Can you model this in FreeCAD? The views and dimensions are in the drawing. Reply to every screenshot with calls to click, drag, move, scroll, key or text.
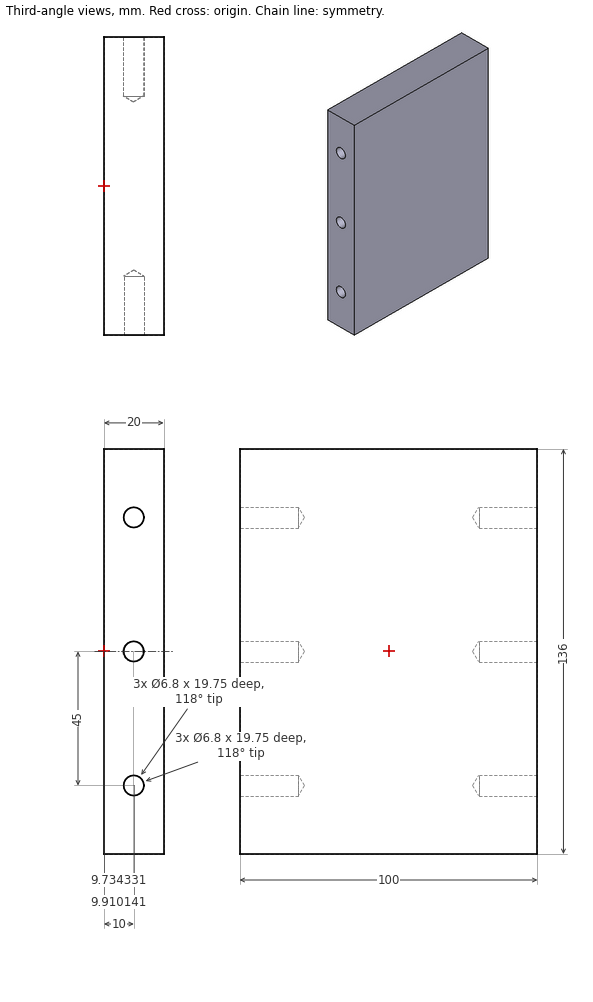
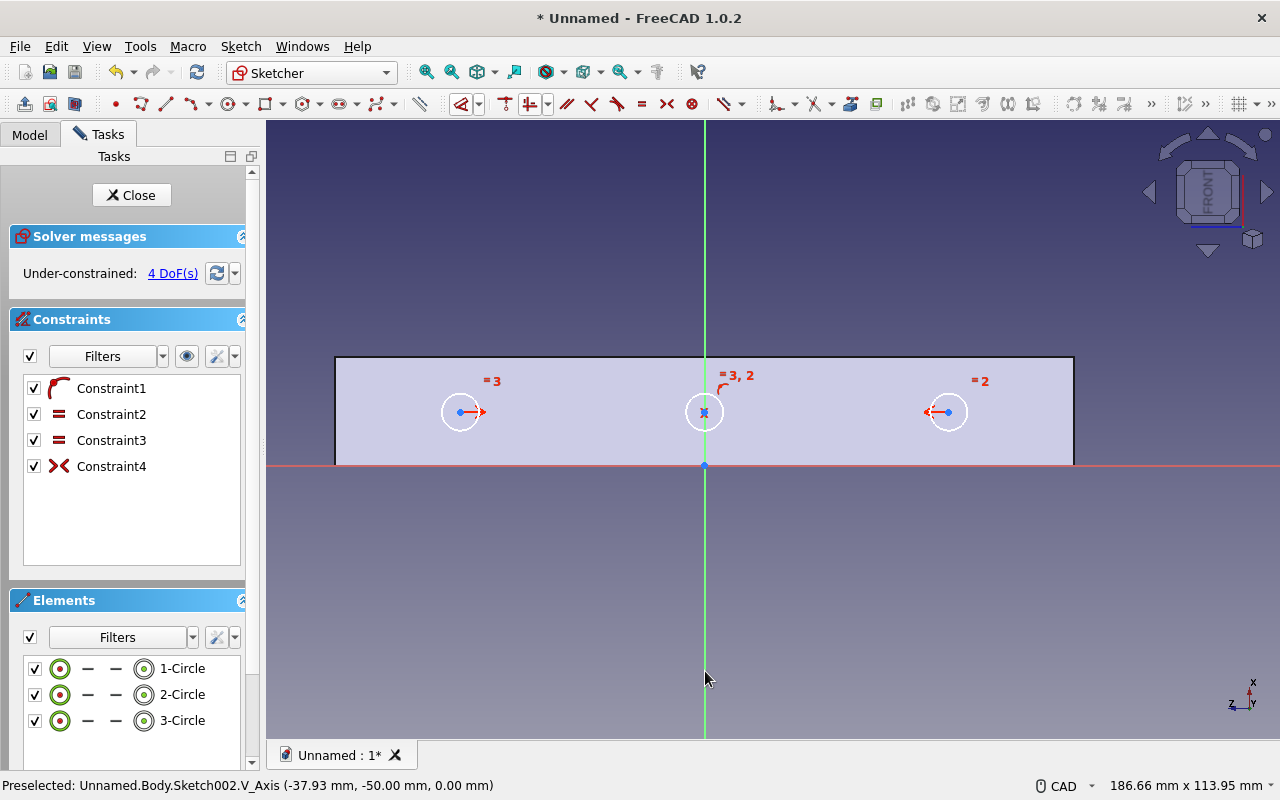
click(962, 399)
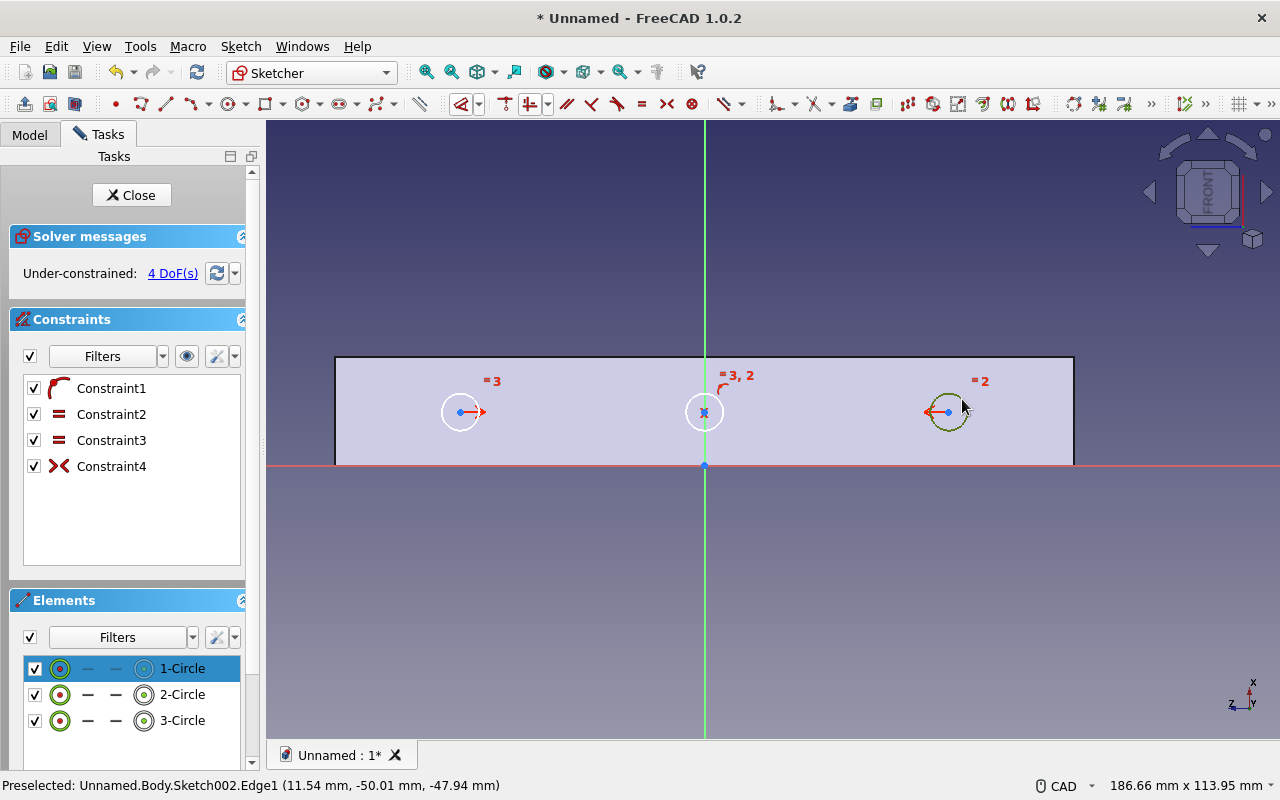
key(k)
key(o)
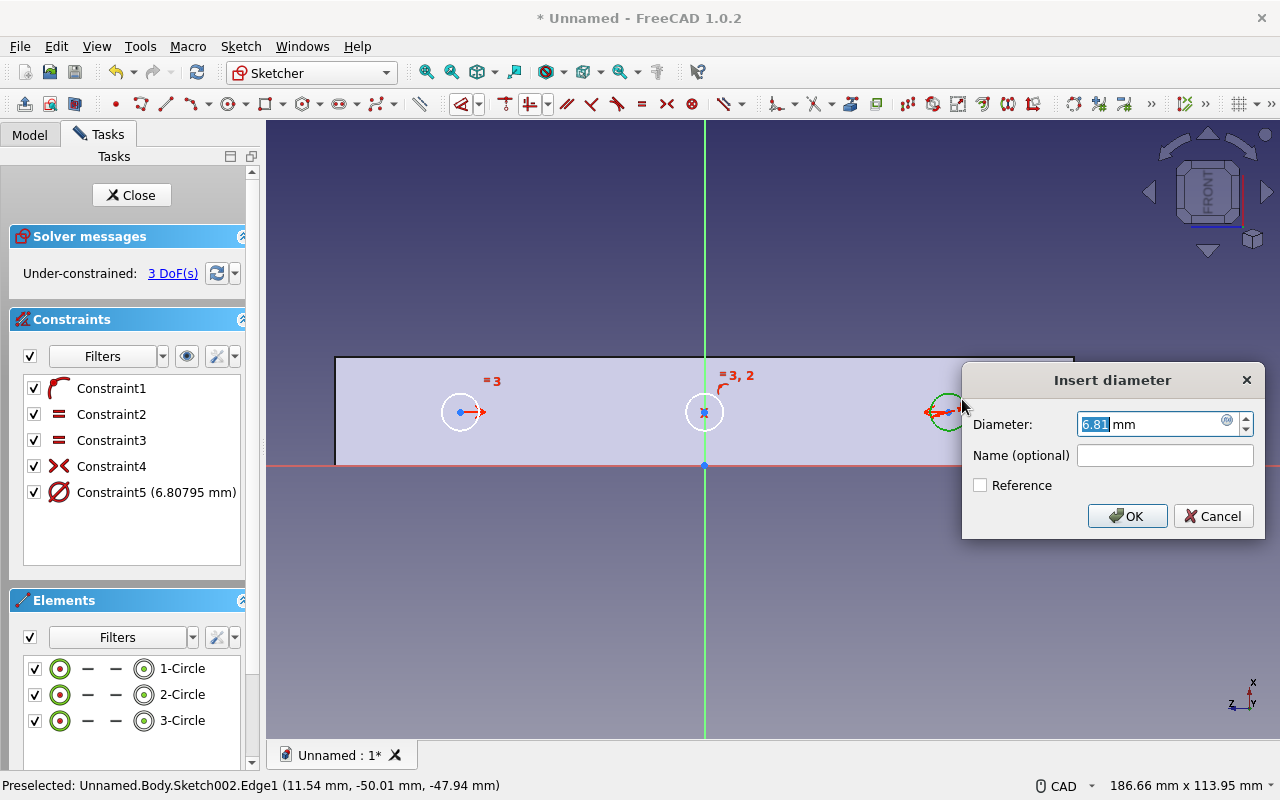
text(6.8)
key(Return)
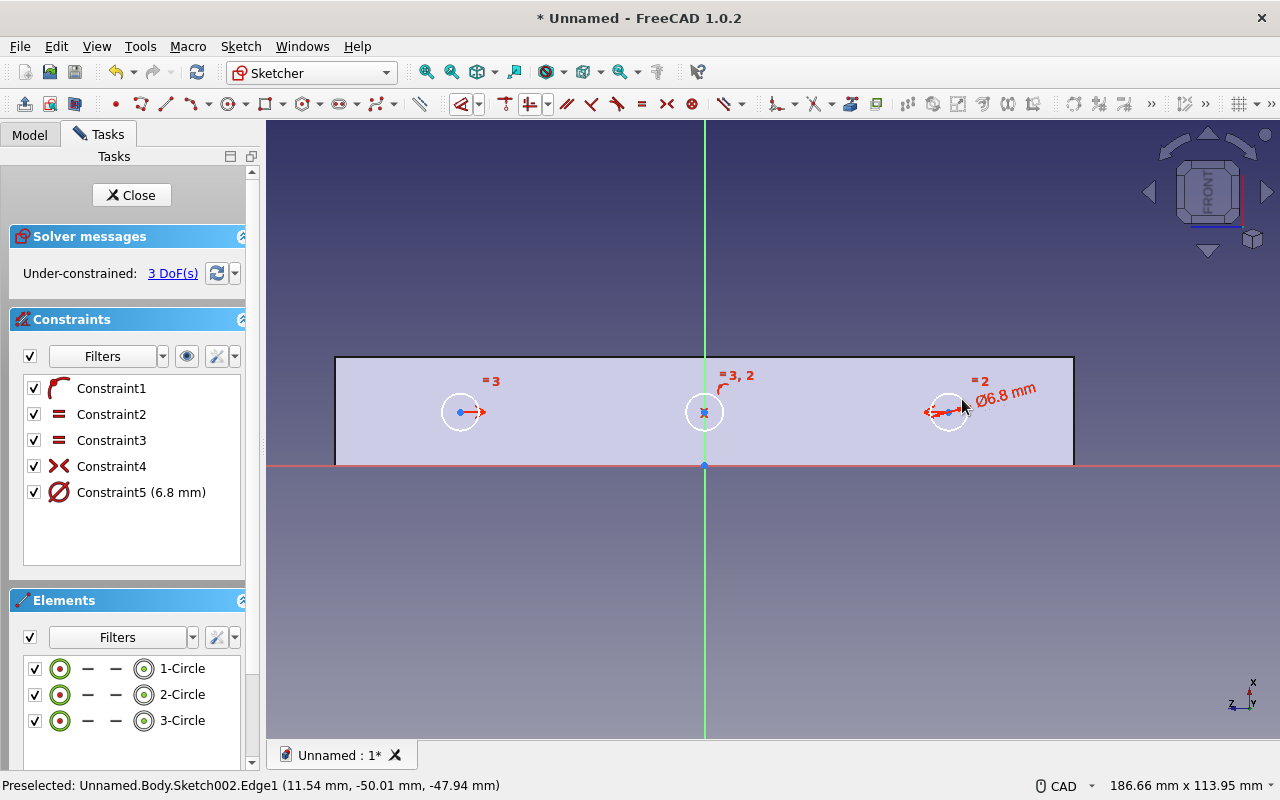
click(949, 412)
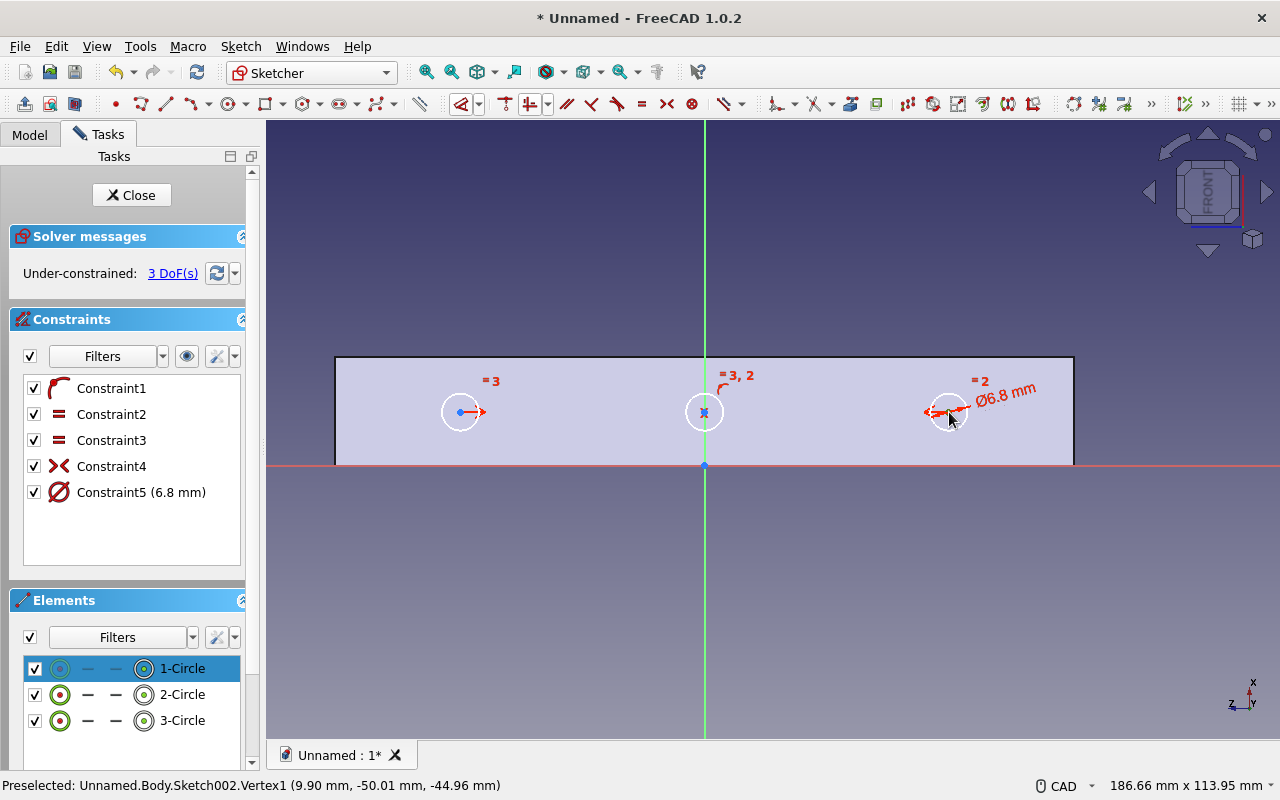
click(478, 104)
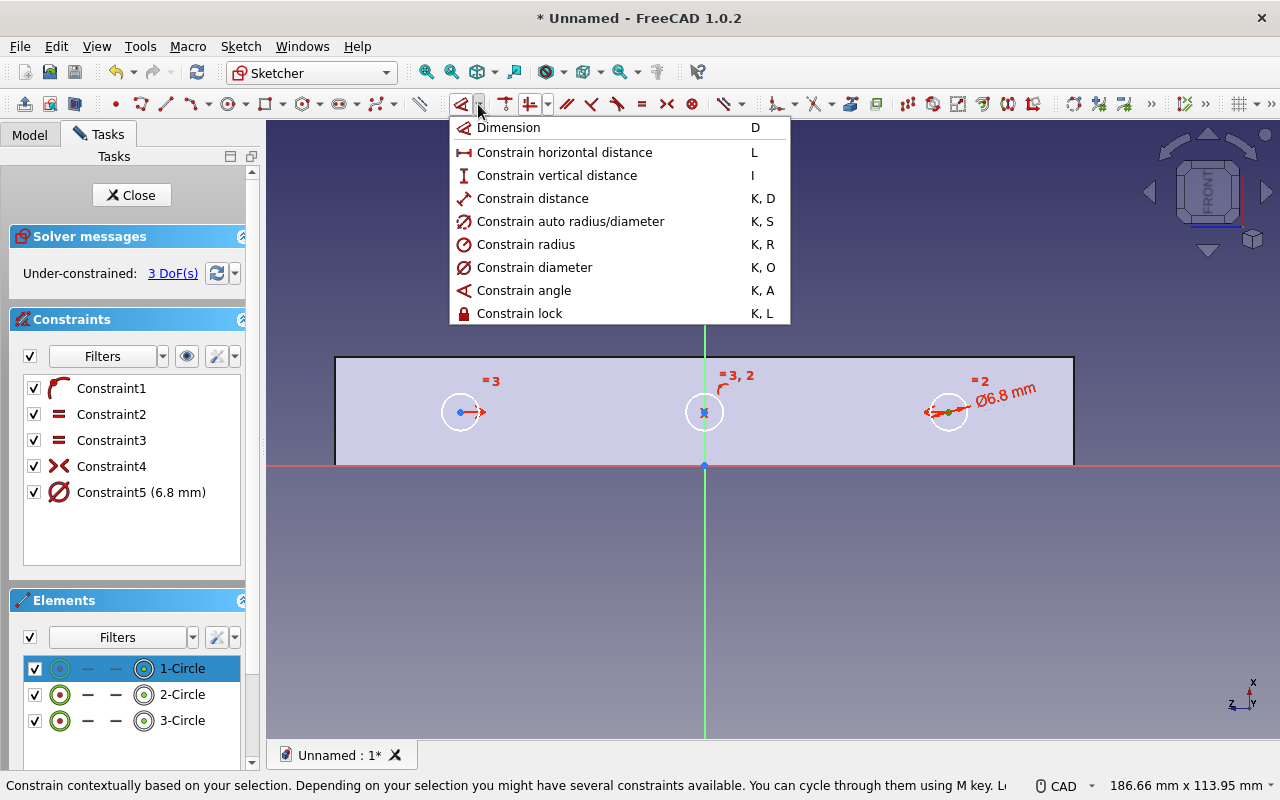
click(620, 152)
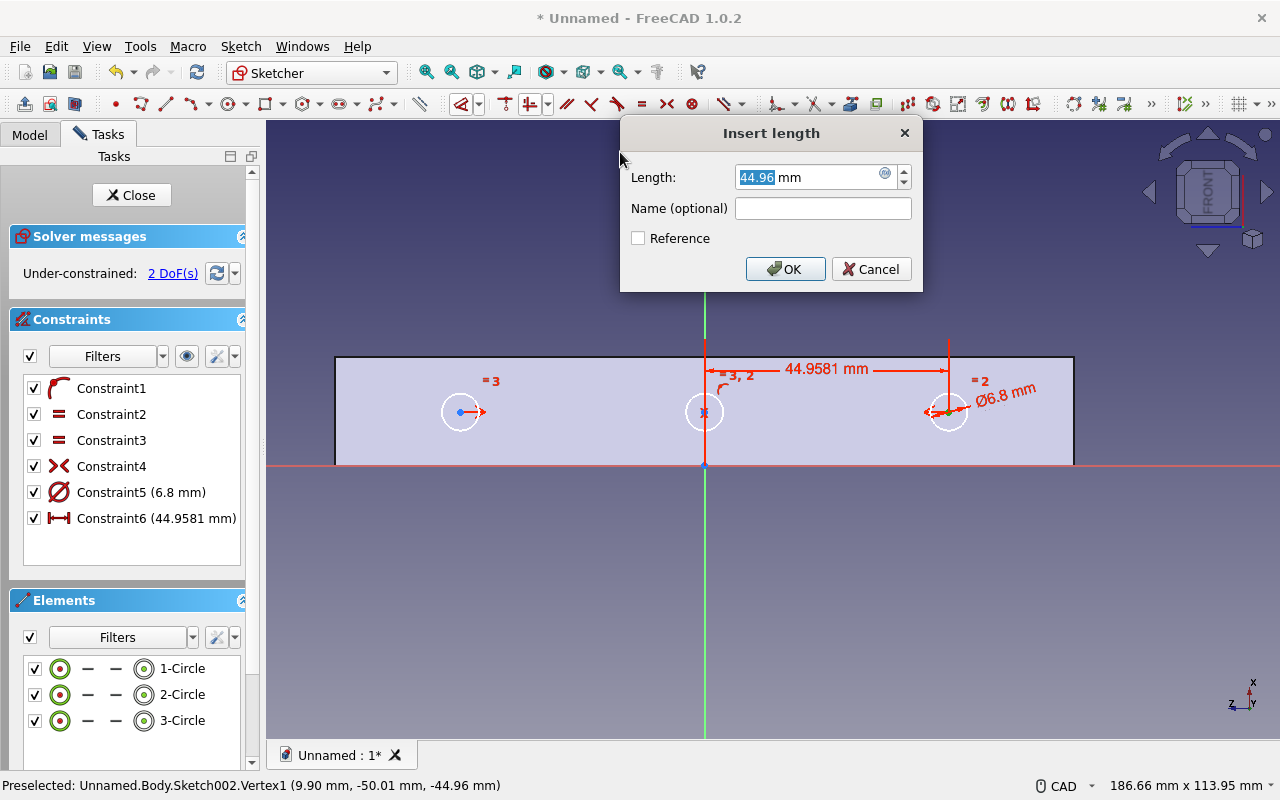
text(45)
key(Return)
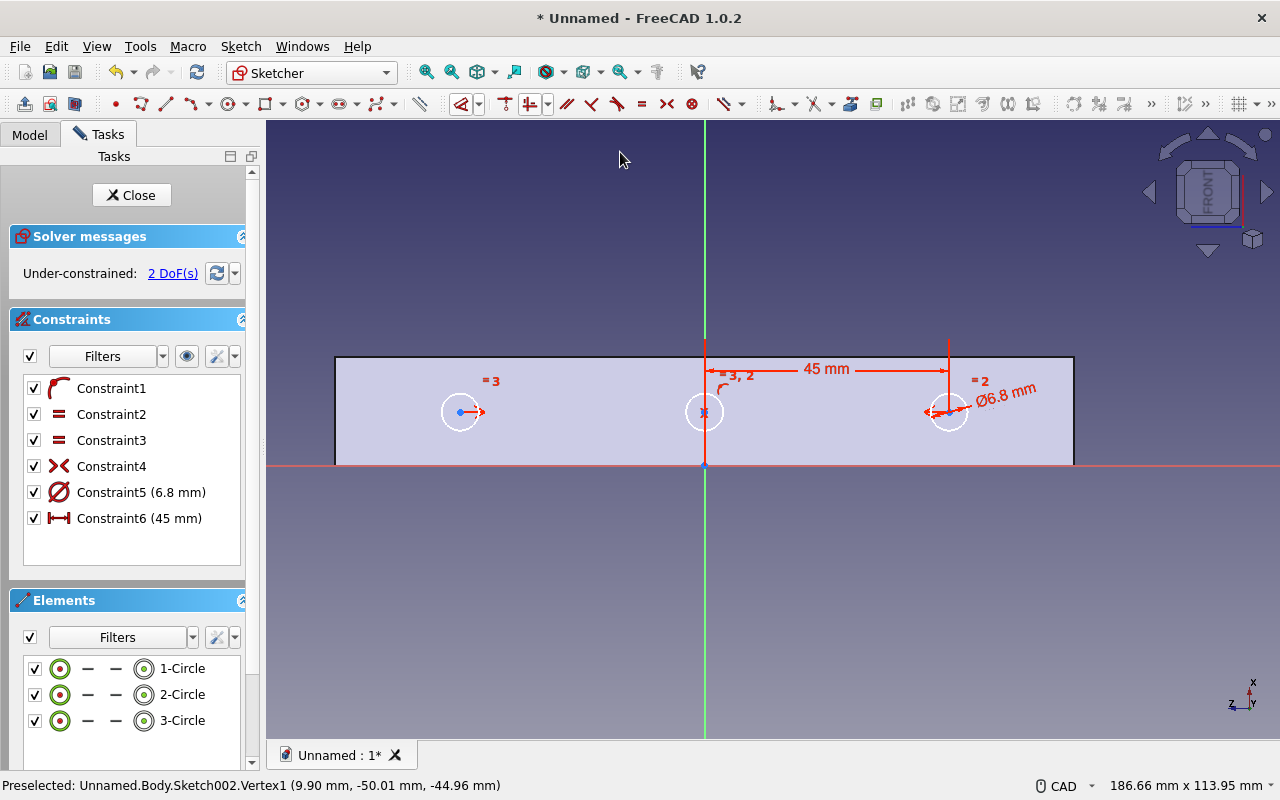
click(949, 412)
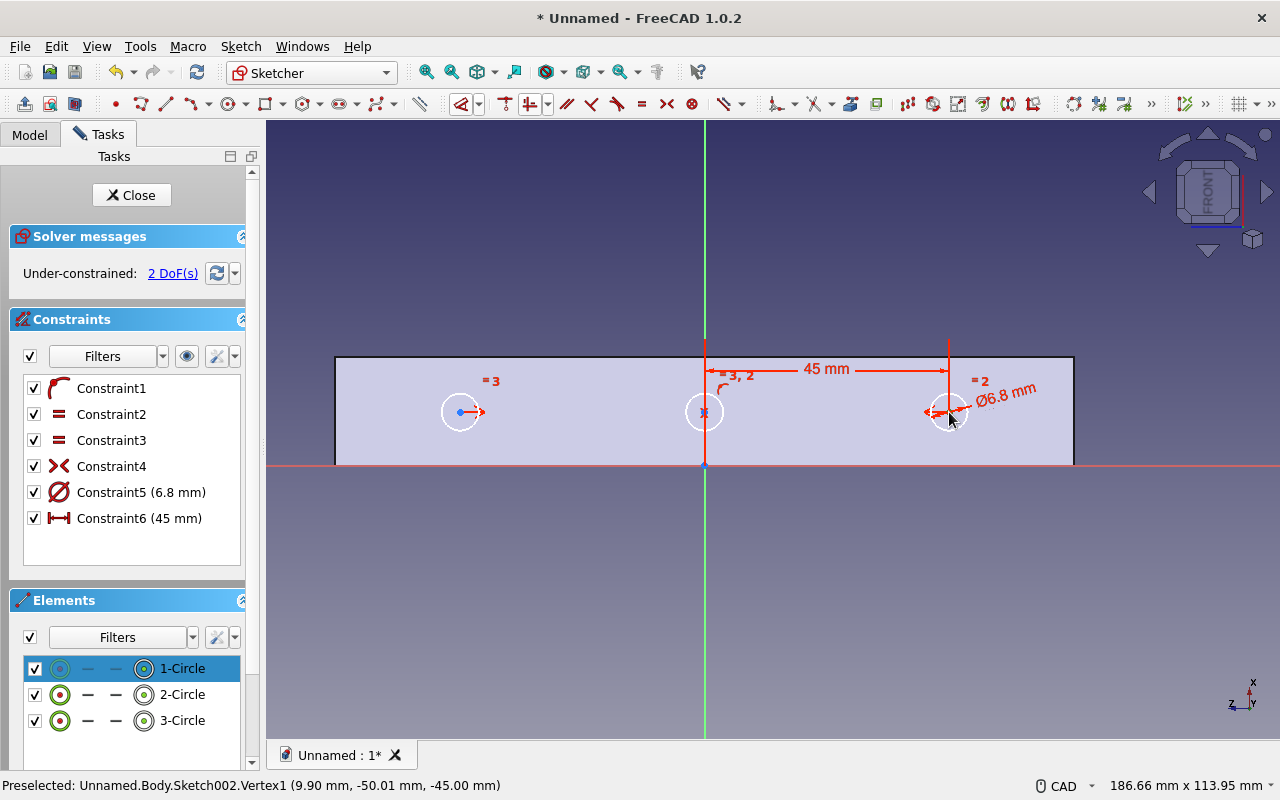
key(i)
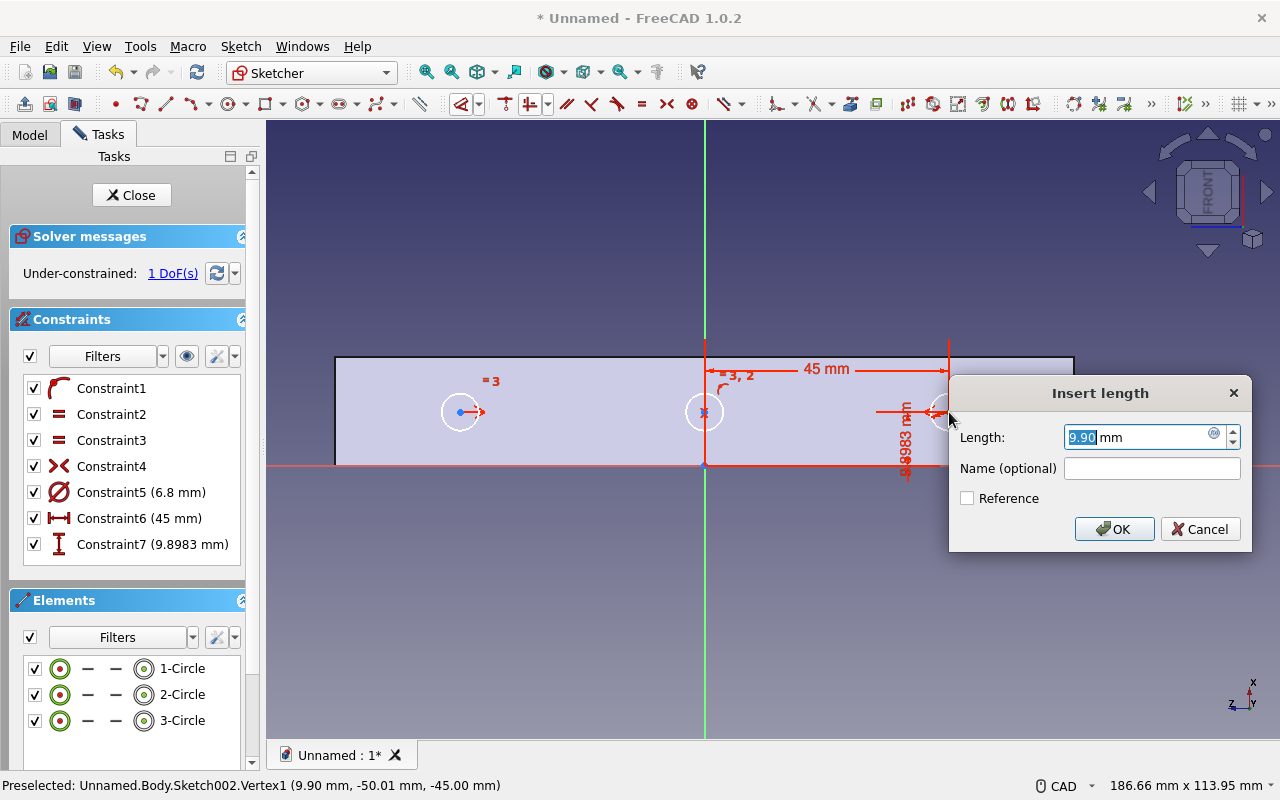
text(10)
key(Return)